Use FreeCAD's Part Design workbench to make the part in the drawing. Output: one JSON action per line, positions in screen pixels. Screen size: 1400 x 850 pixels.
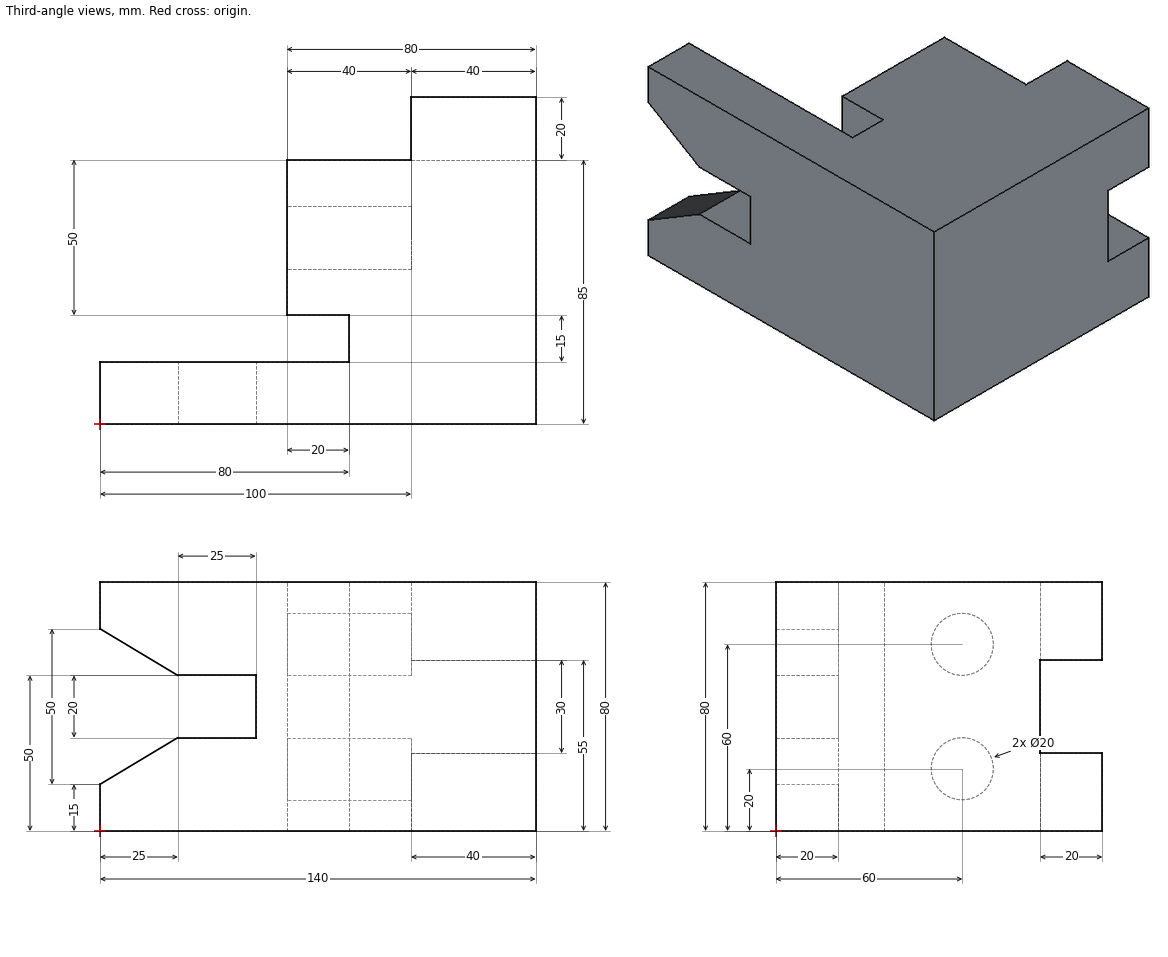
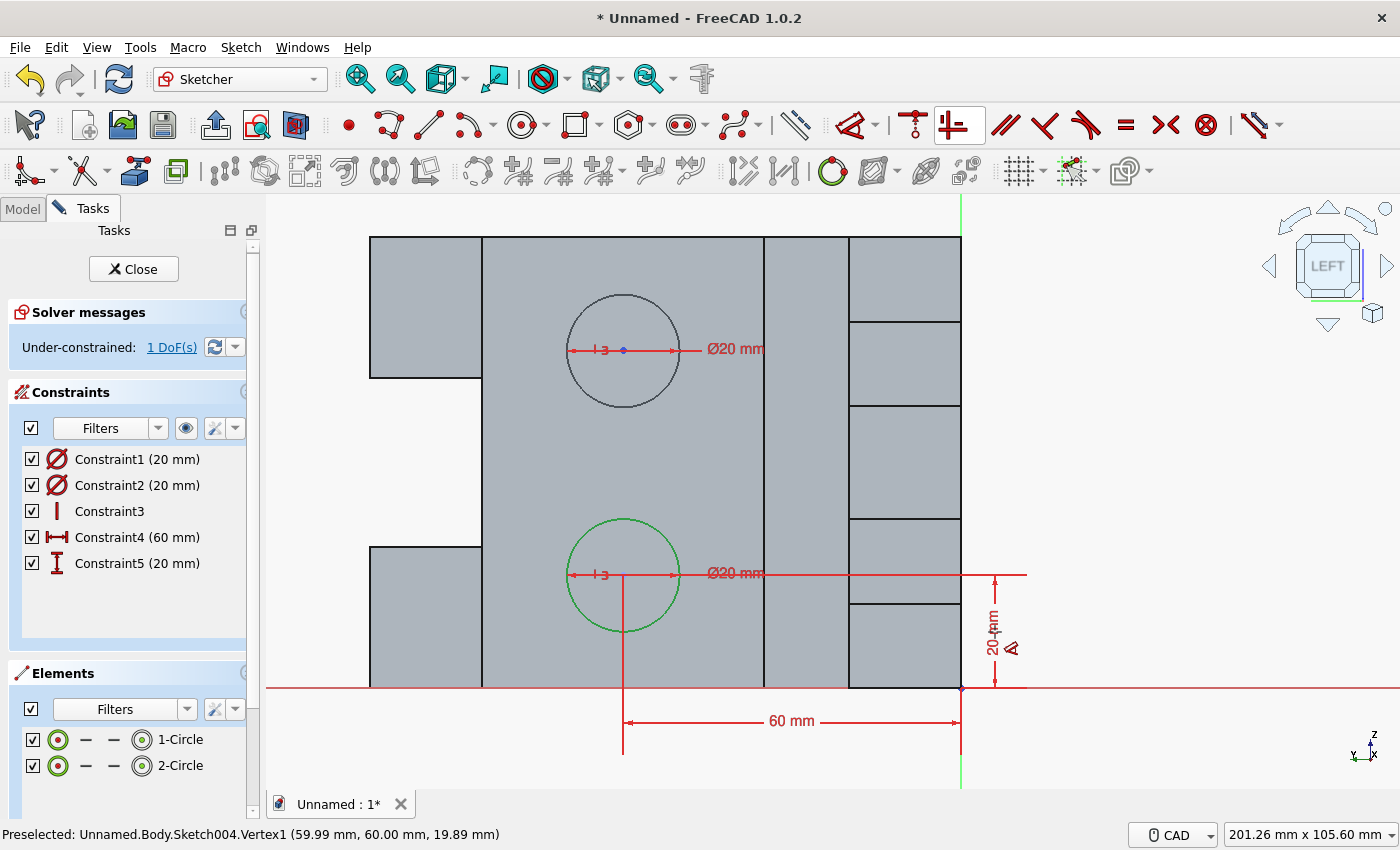
{"action": "left_click", "coordinate": [623, 351]}
{"action": "left_click", "coordinate": [995, 520]}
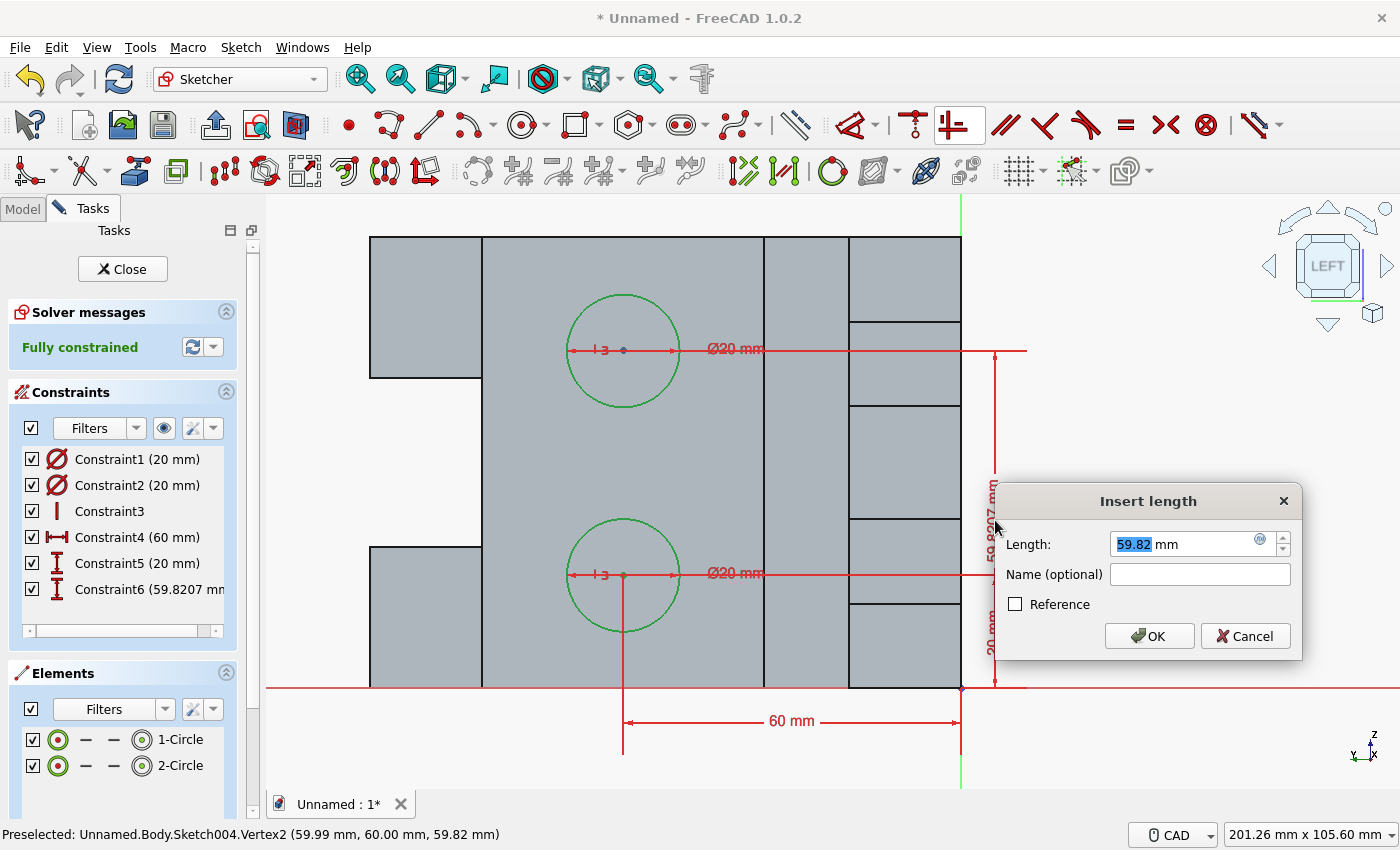
{"action": "type", "text": "60"}
{"action": "key", "text": "Return"}
{"action": "key", "text": "Escape"}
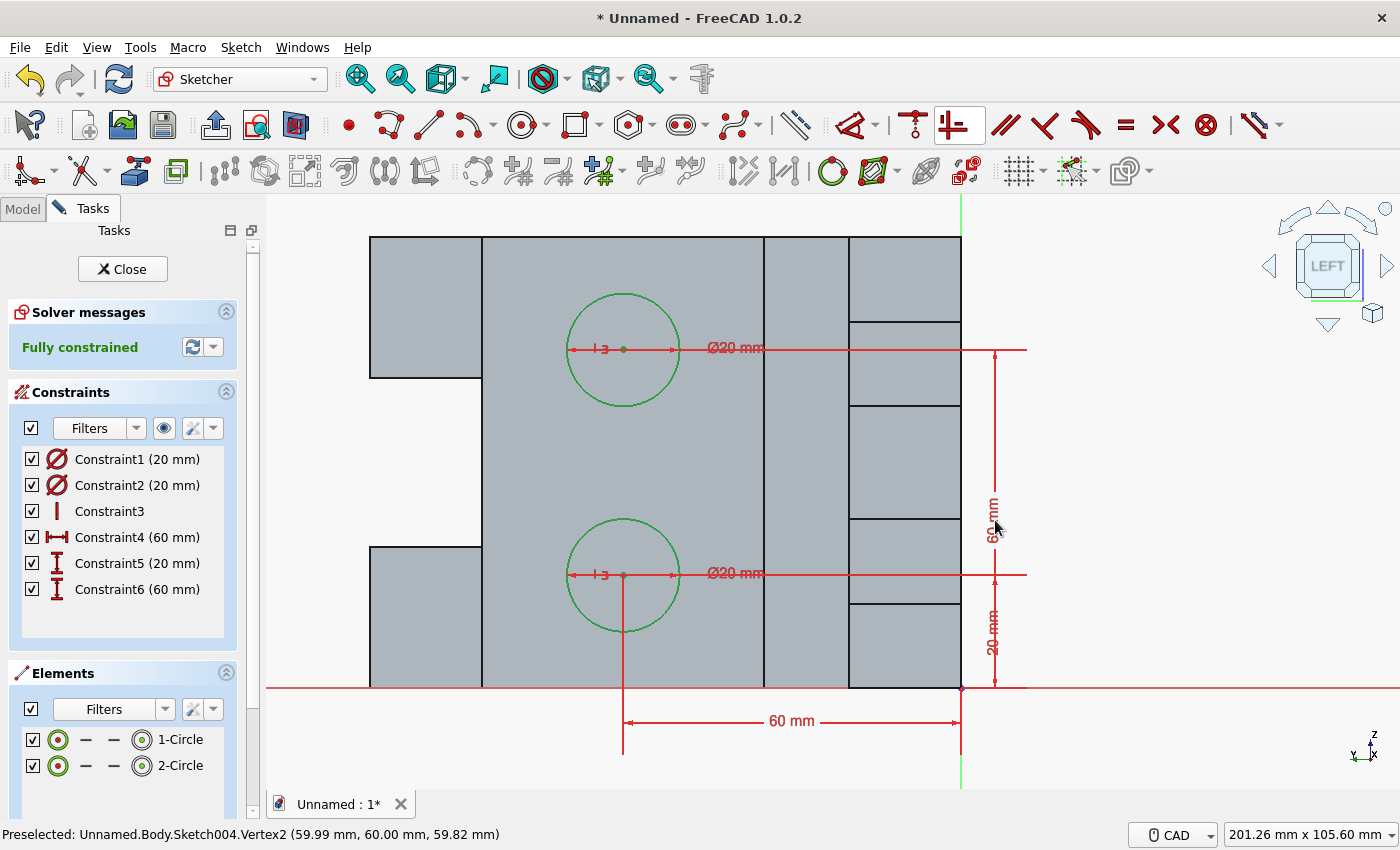
{"action": "left_click", "coordinate": [123, 269]}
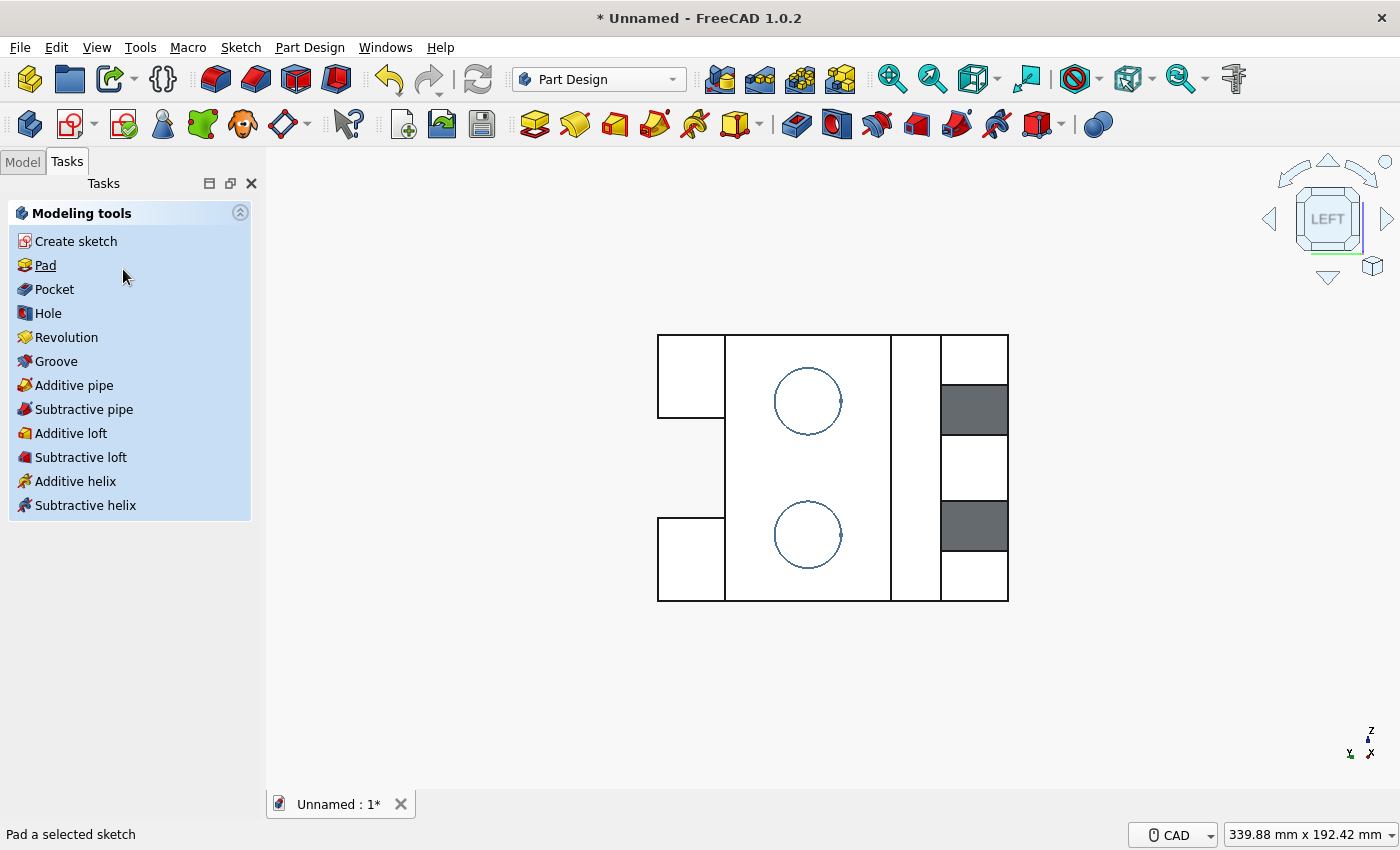
{"action": "left_click", "coordinate": [798, 124]}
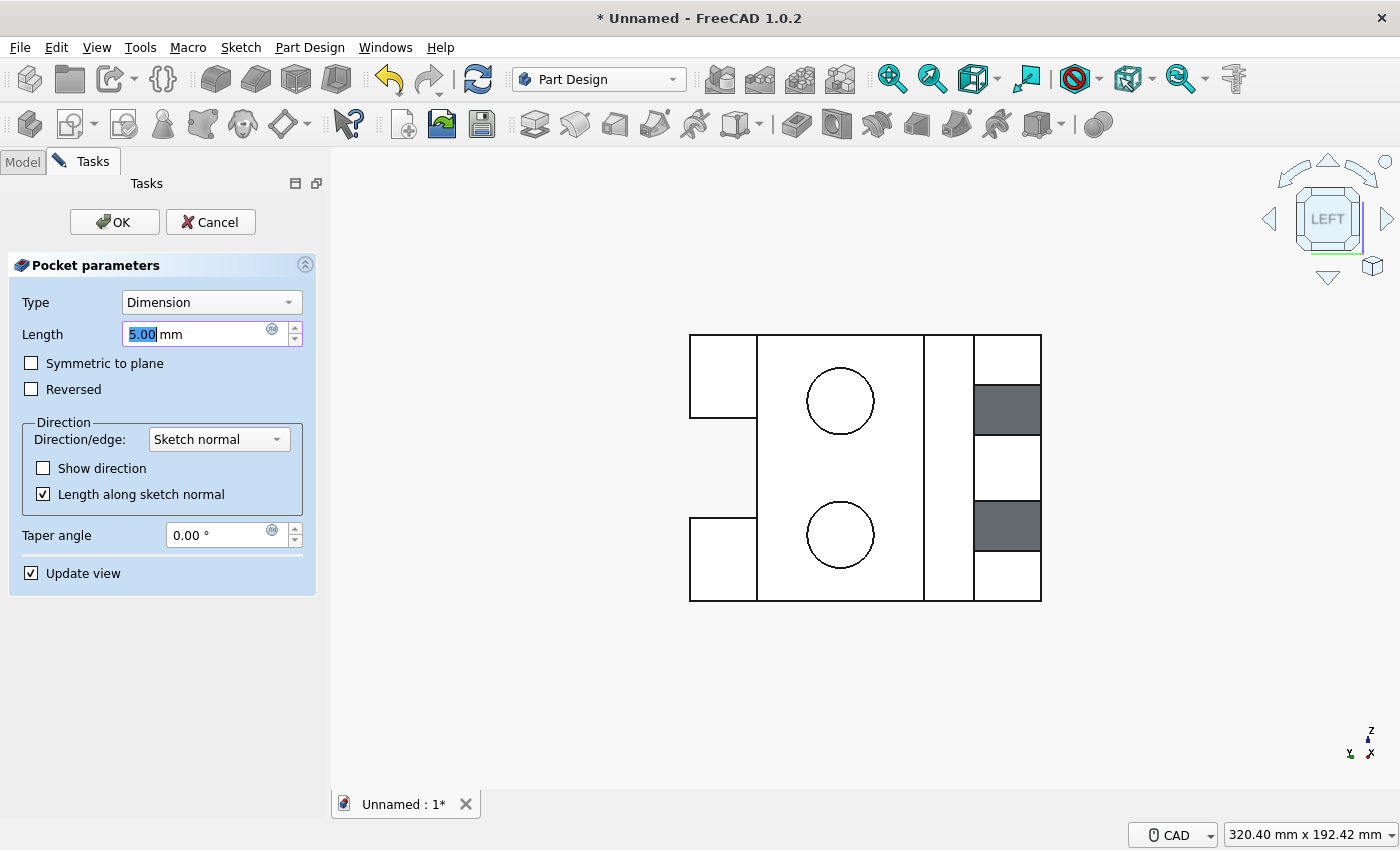
{"action": "type", "text": "40"}
{"action": "key", "text": "Tab"}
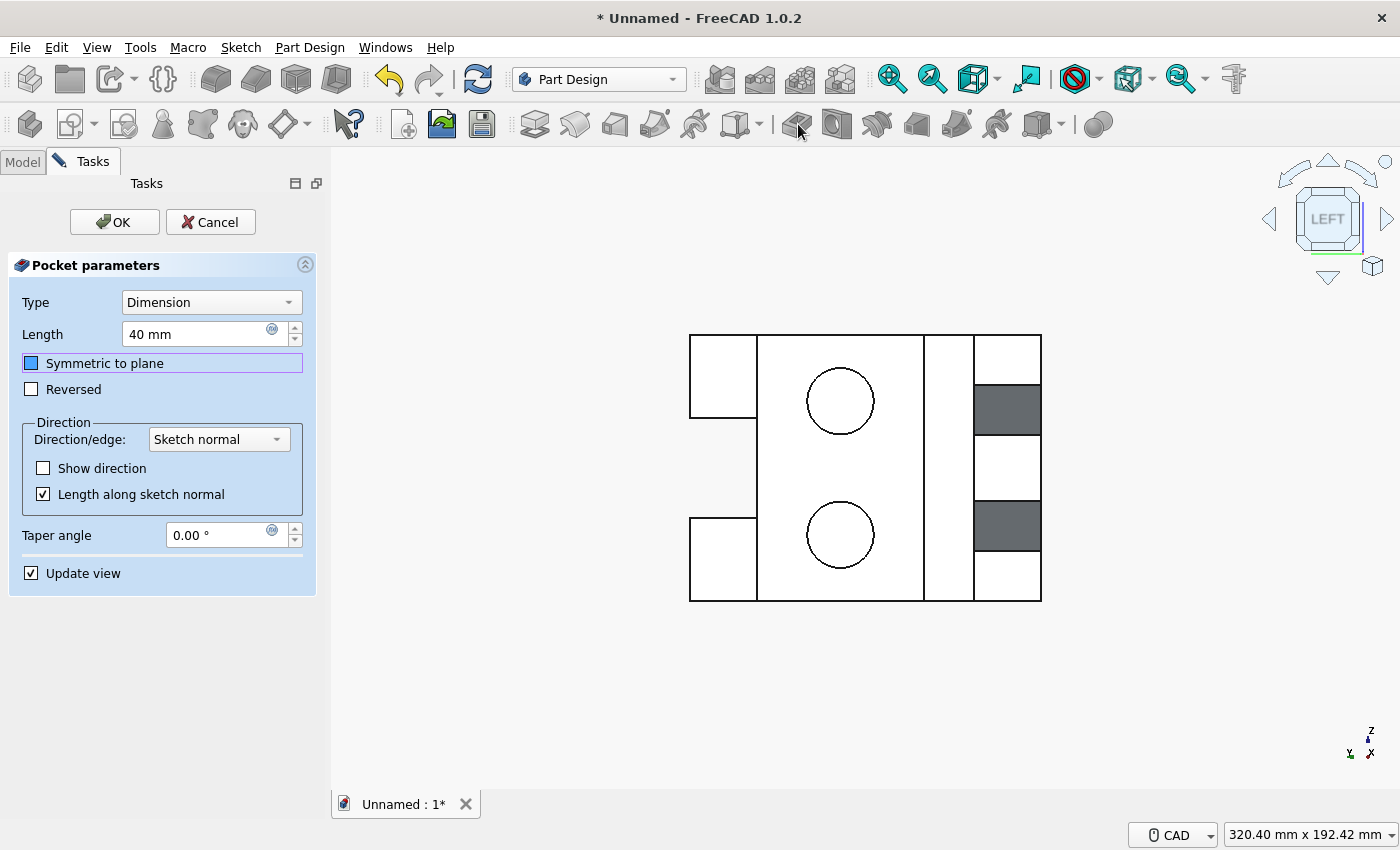
{"action": "left_click", "coordinate": [115, 222]}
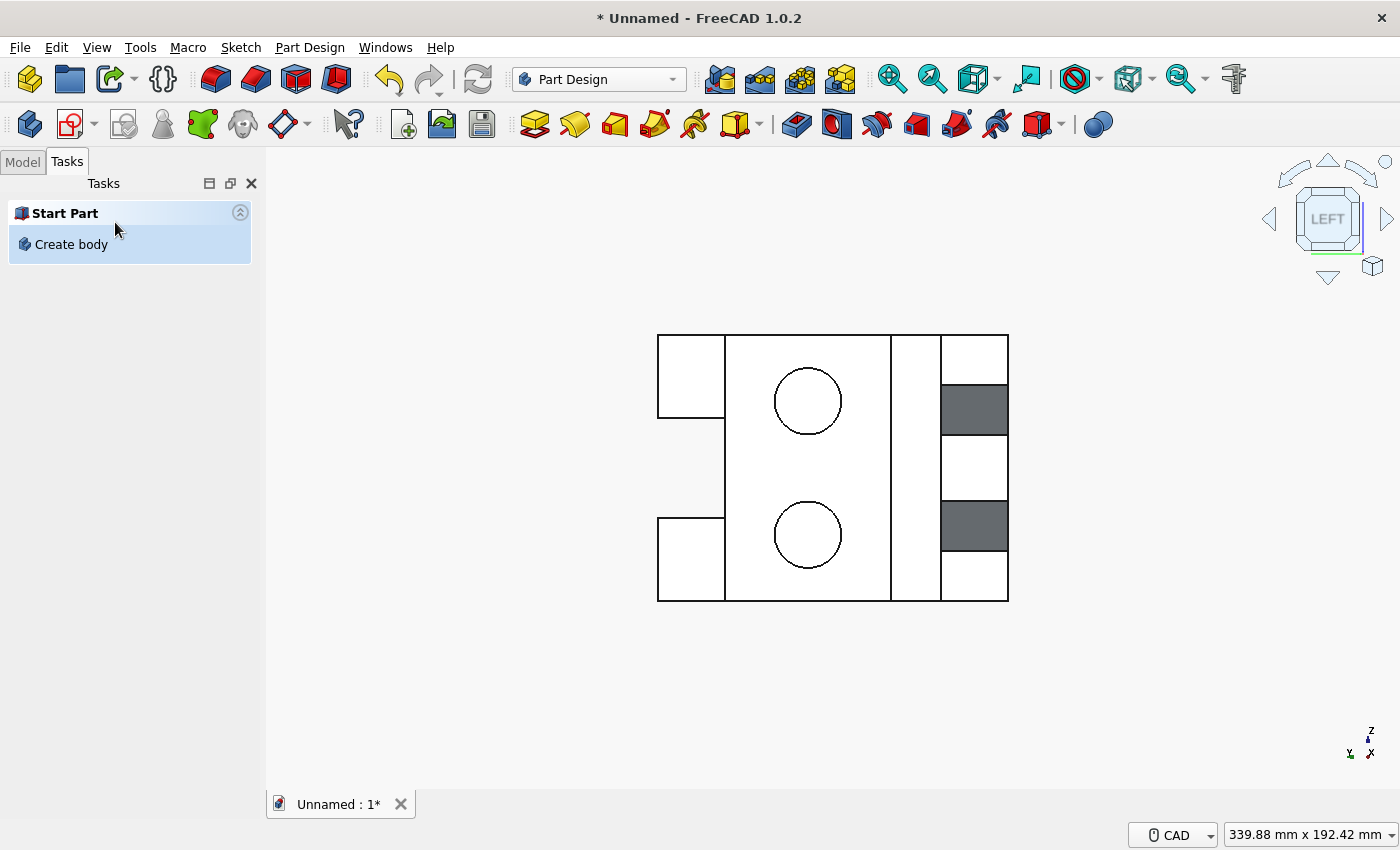
{"action": "key", "text": "0"}